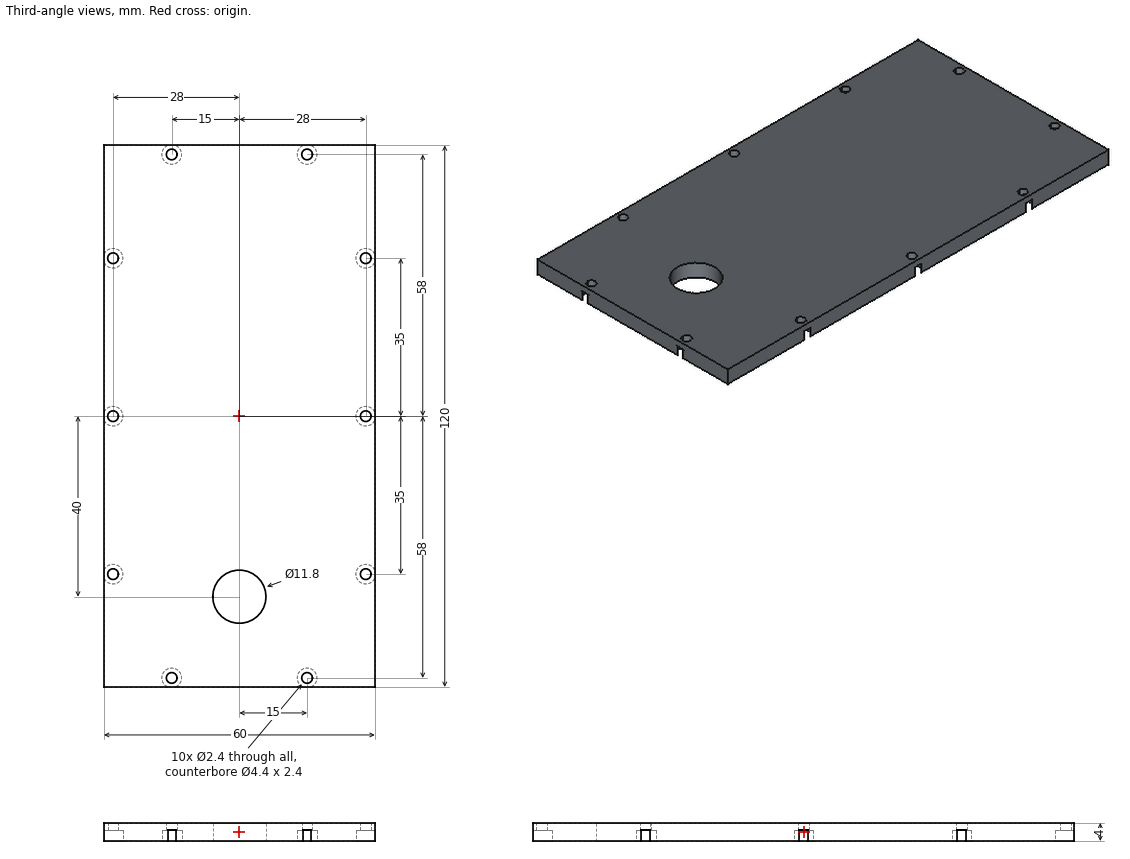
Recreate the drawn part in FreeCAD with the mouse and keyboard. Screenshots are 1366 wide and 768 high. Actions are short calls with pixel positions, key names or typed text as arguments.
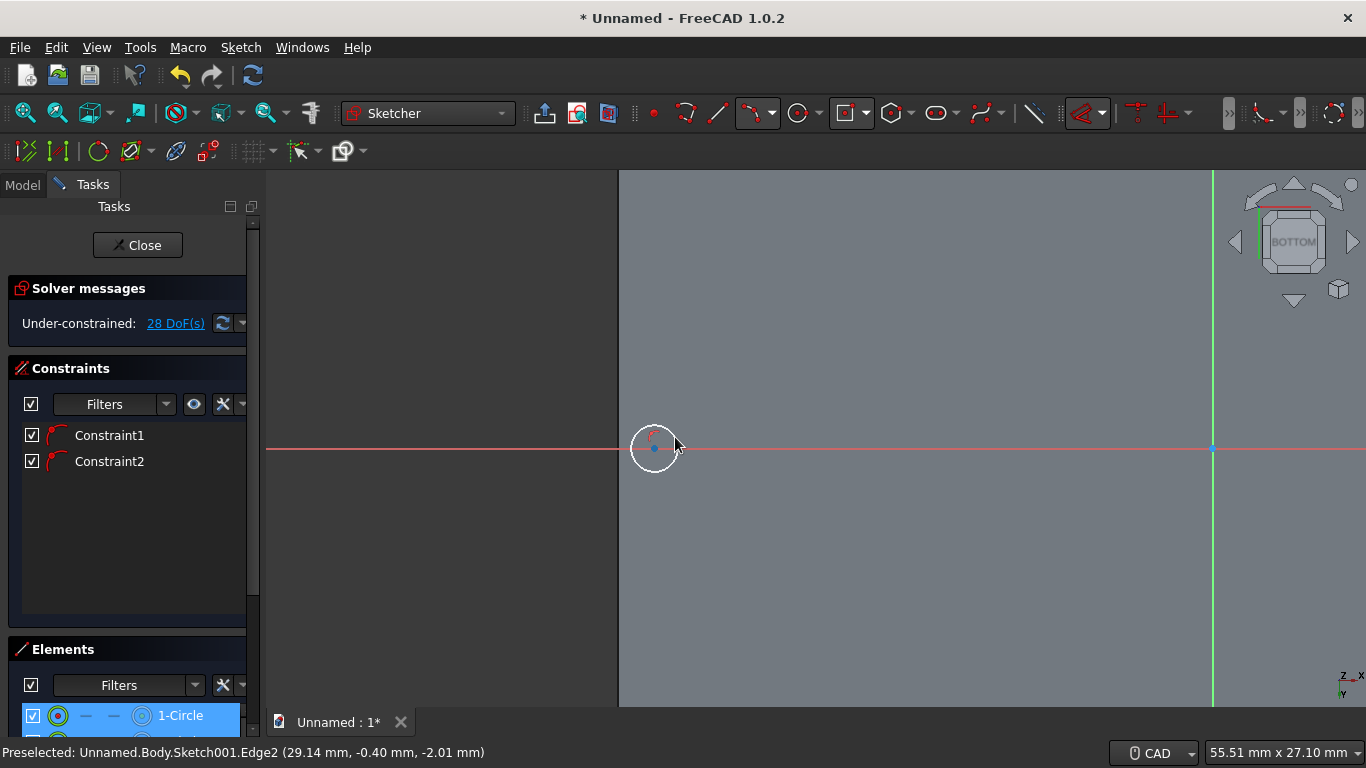
click(671, 432)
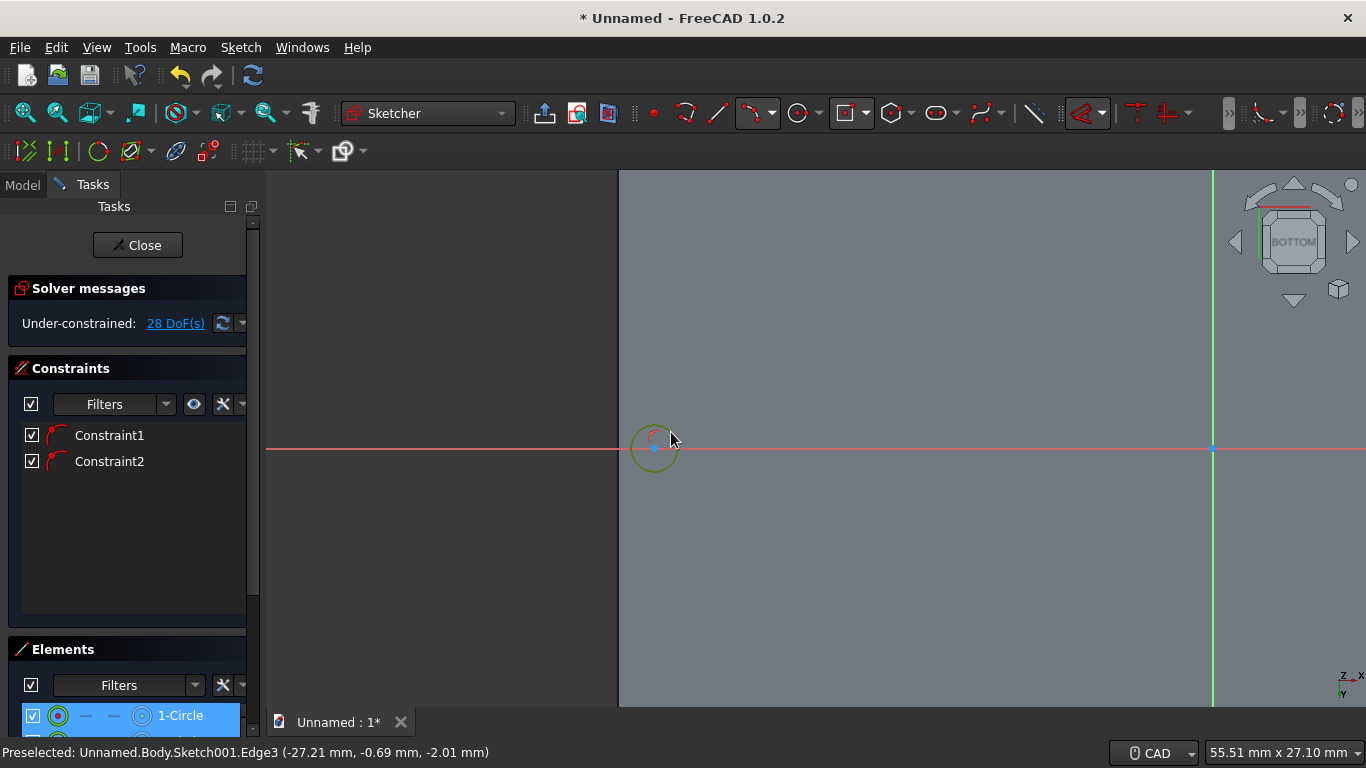
scroll(675, 437, down, 10)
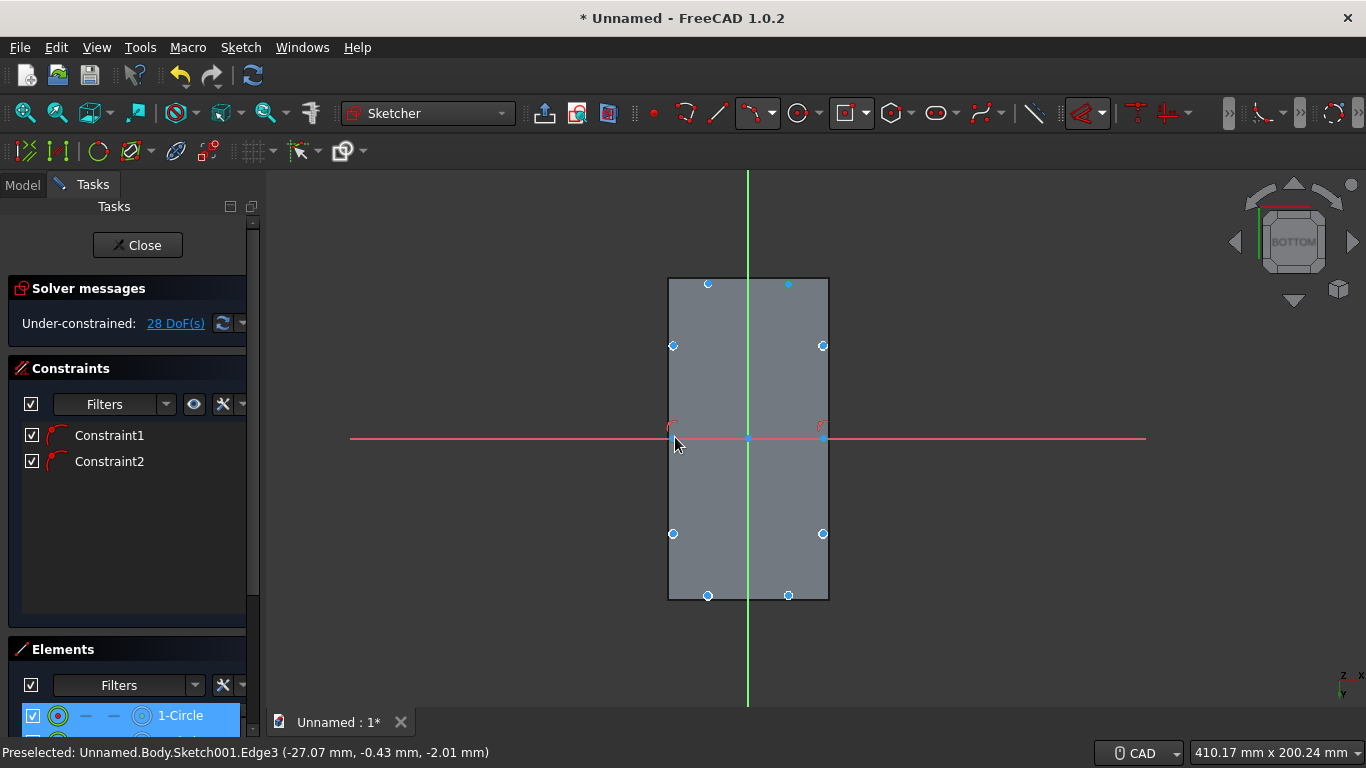
scroll(791, 593, up, 7)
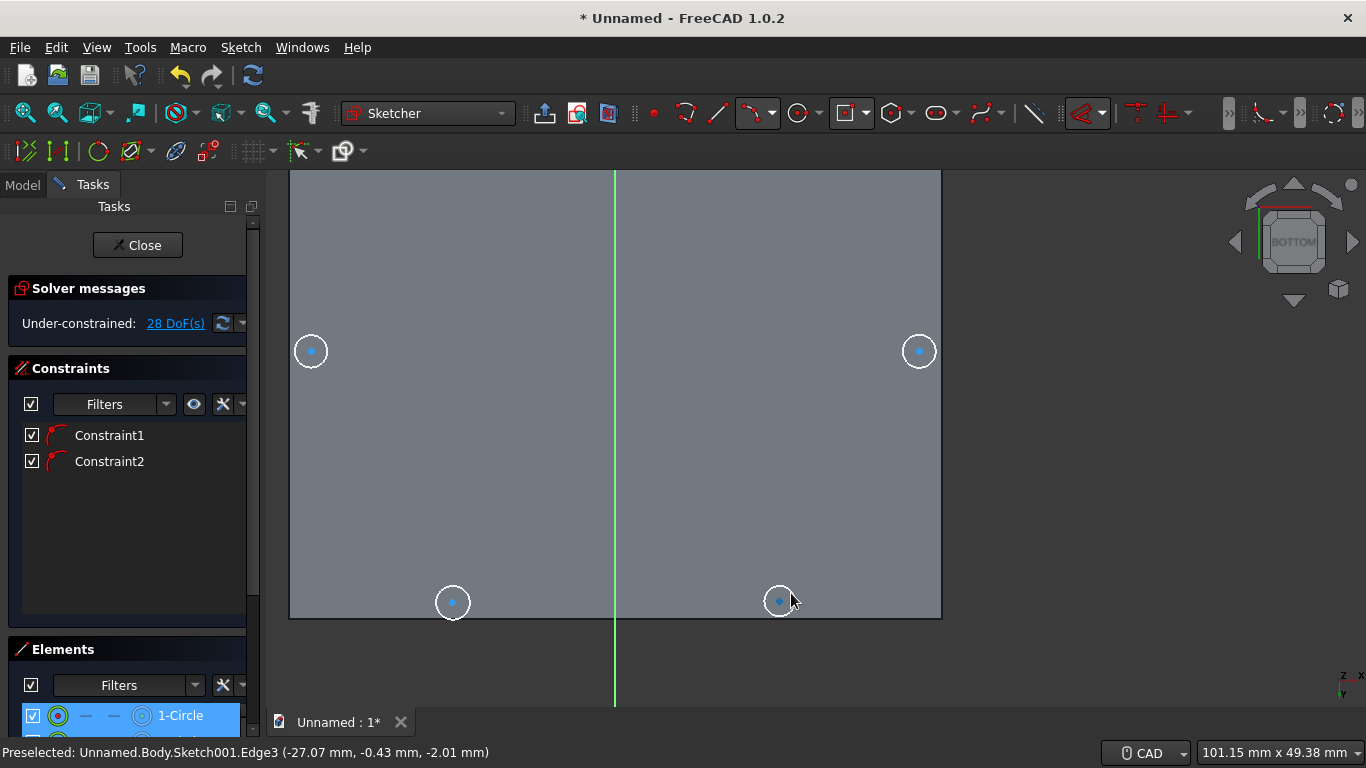
click(790, 590)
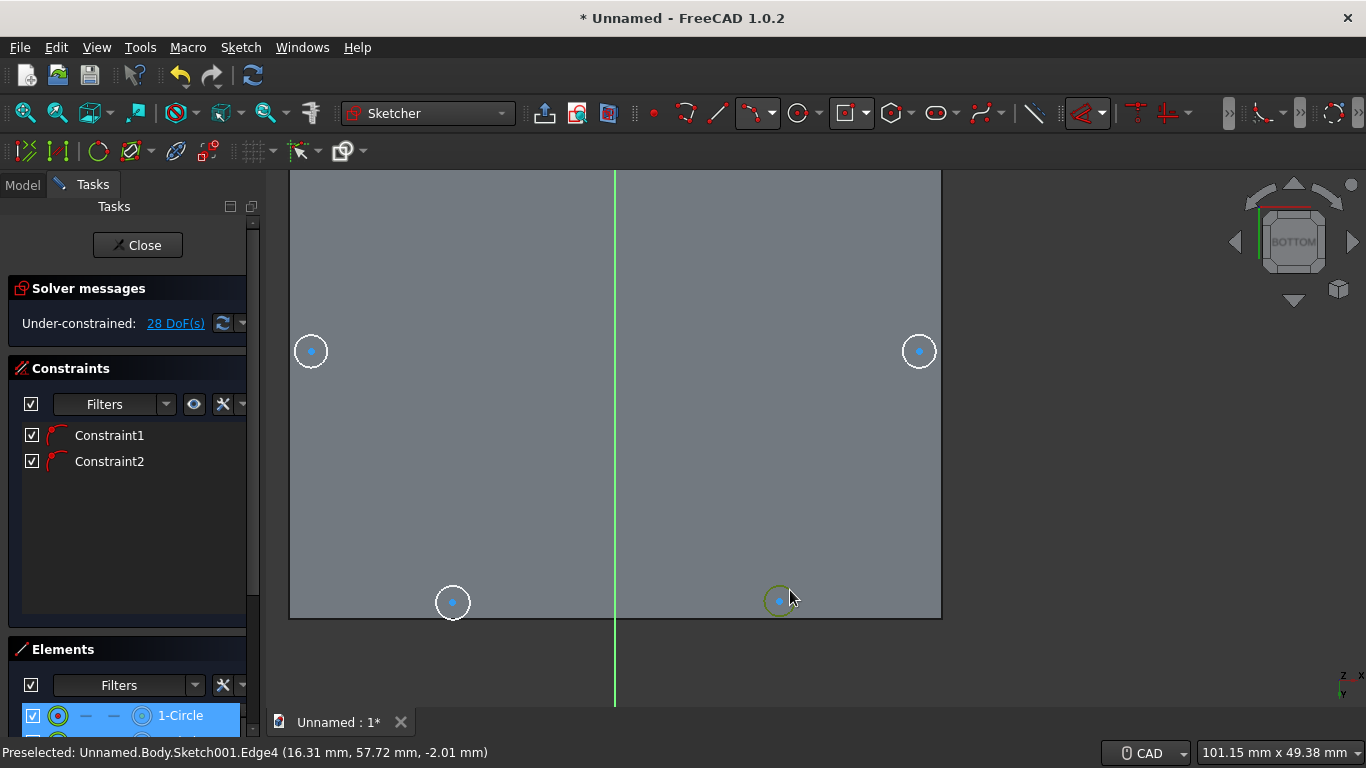
click(465, 591)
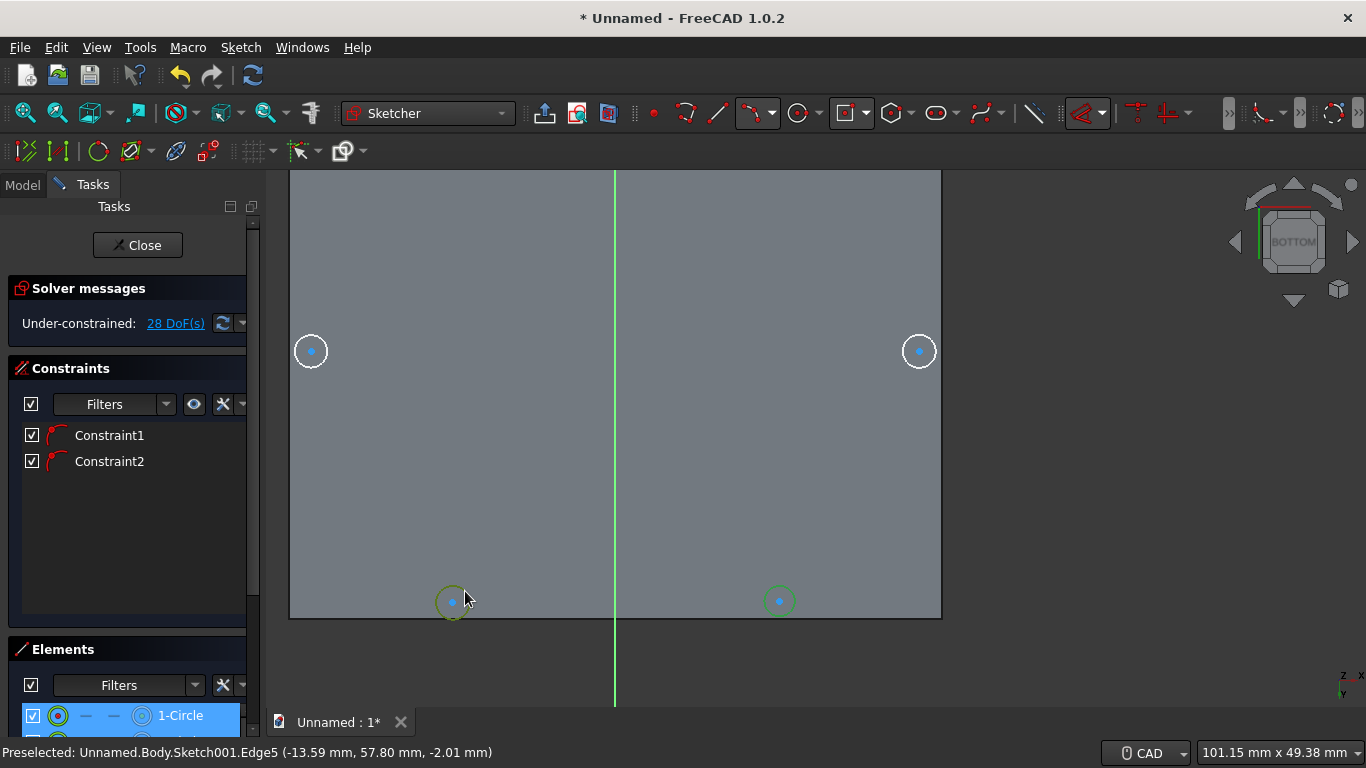
click(931, 340)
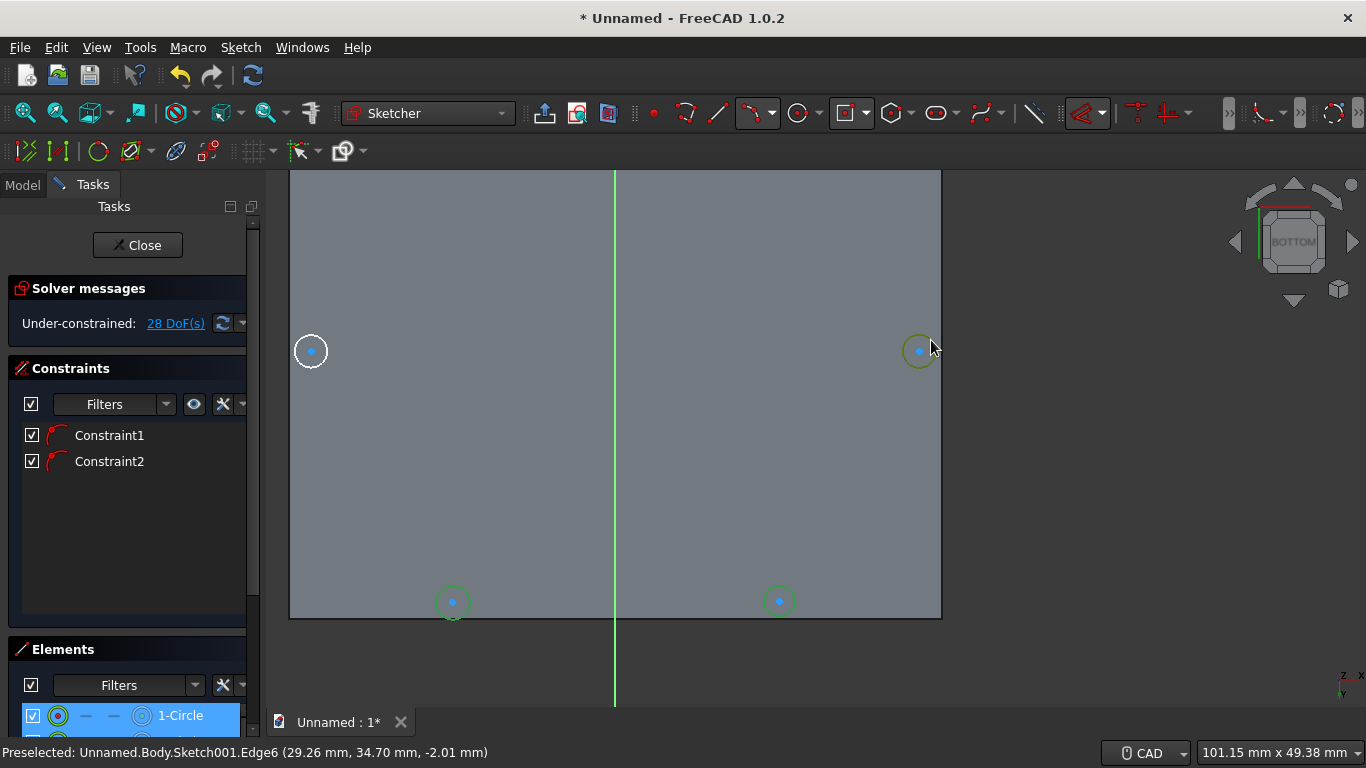
click(322, 340)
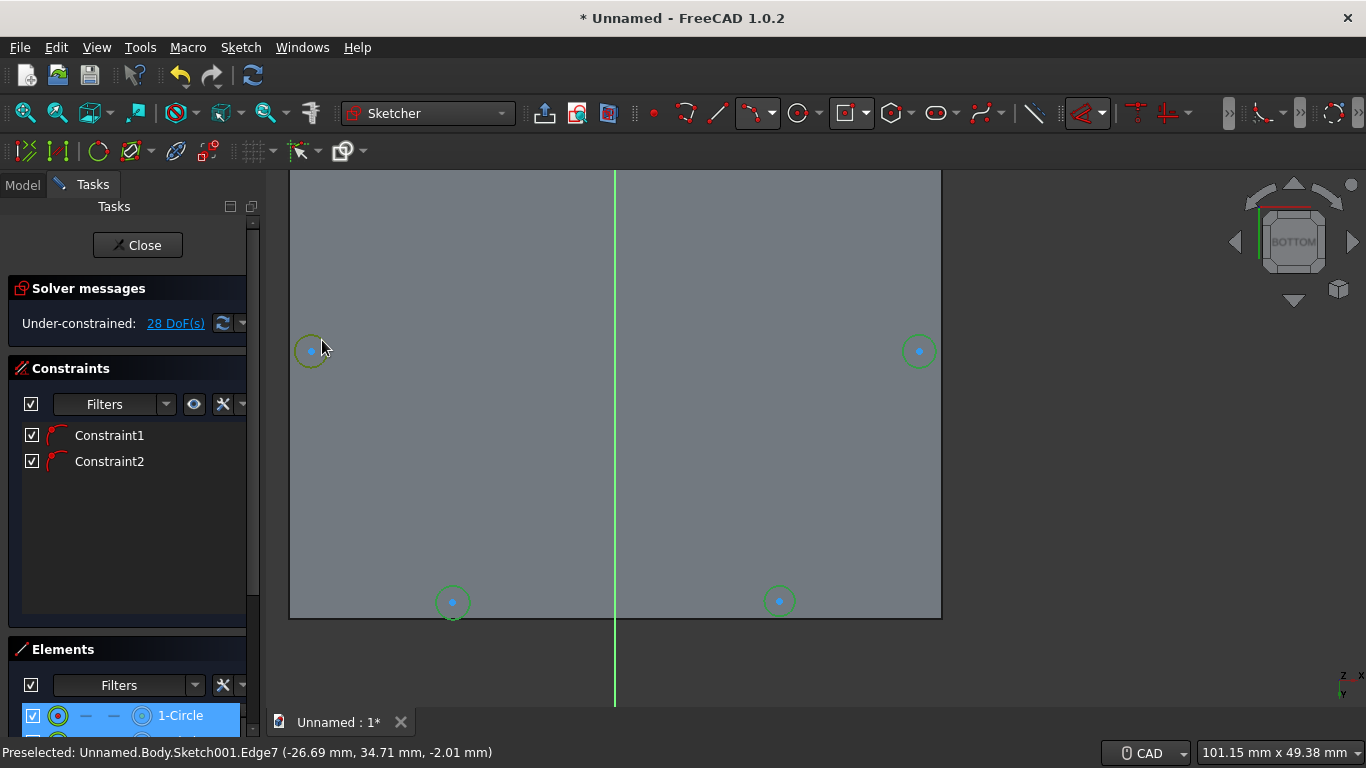
scroll(791, 593, down, 7)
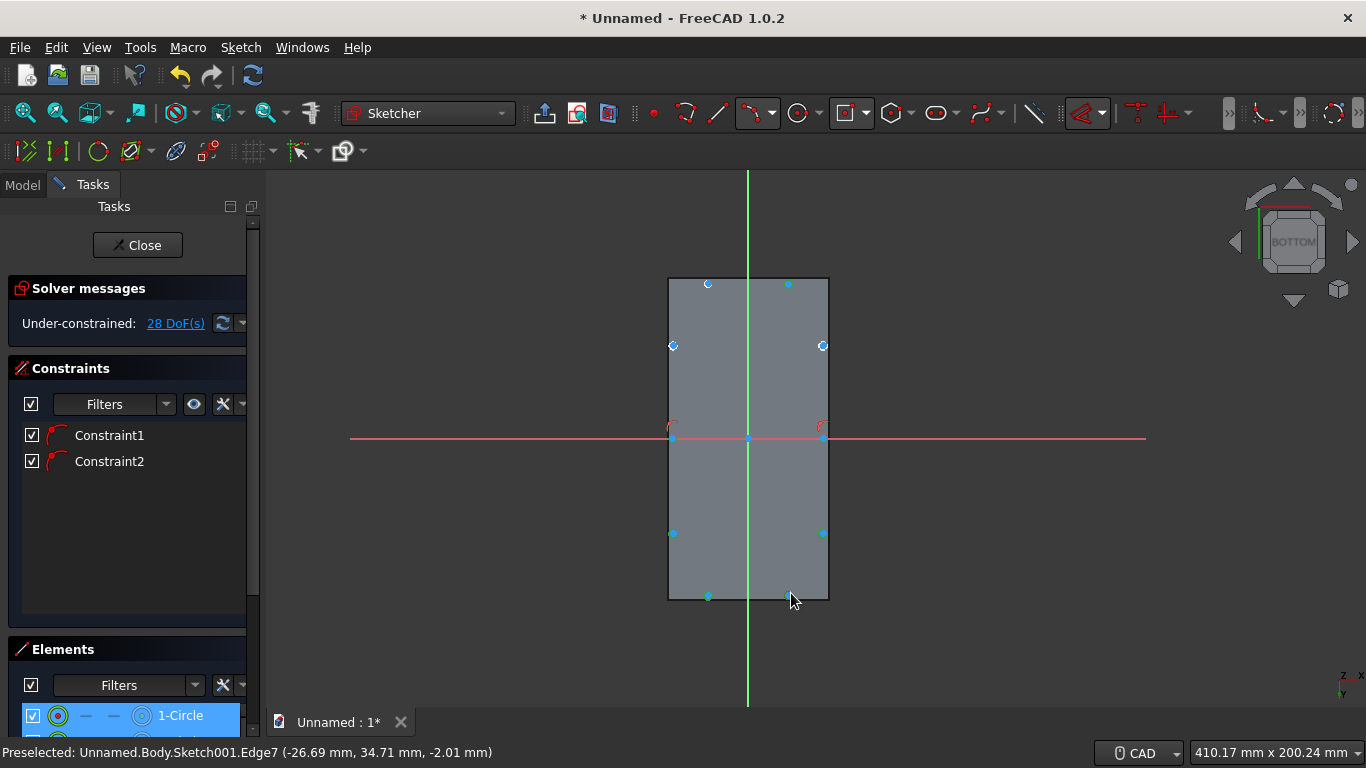
scroll(826, 343, up, 7)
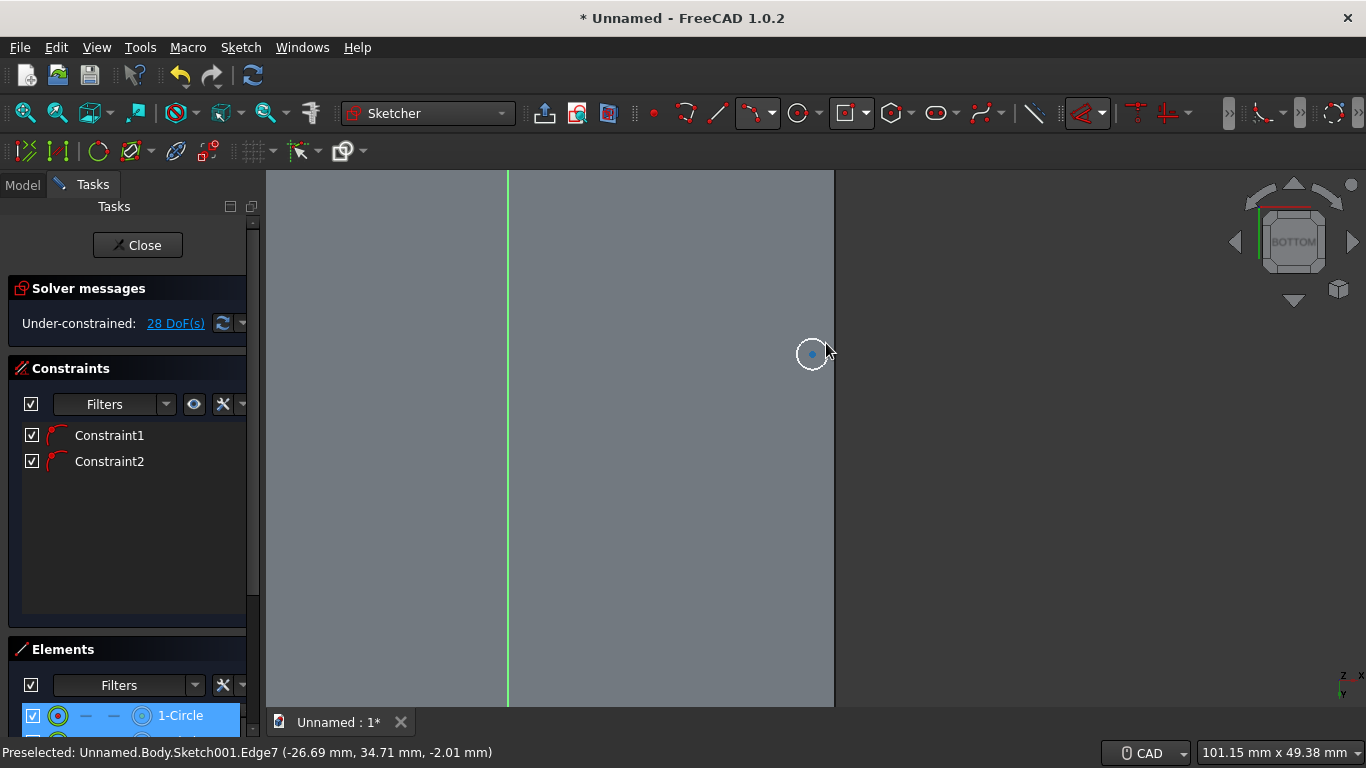
click(823, 343)